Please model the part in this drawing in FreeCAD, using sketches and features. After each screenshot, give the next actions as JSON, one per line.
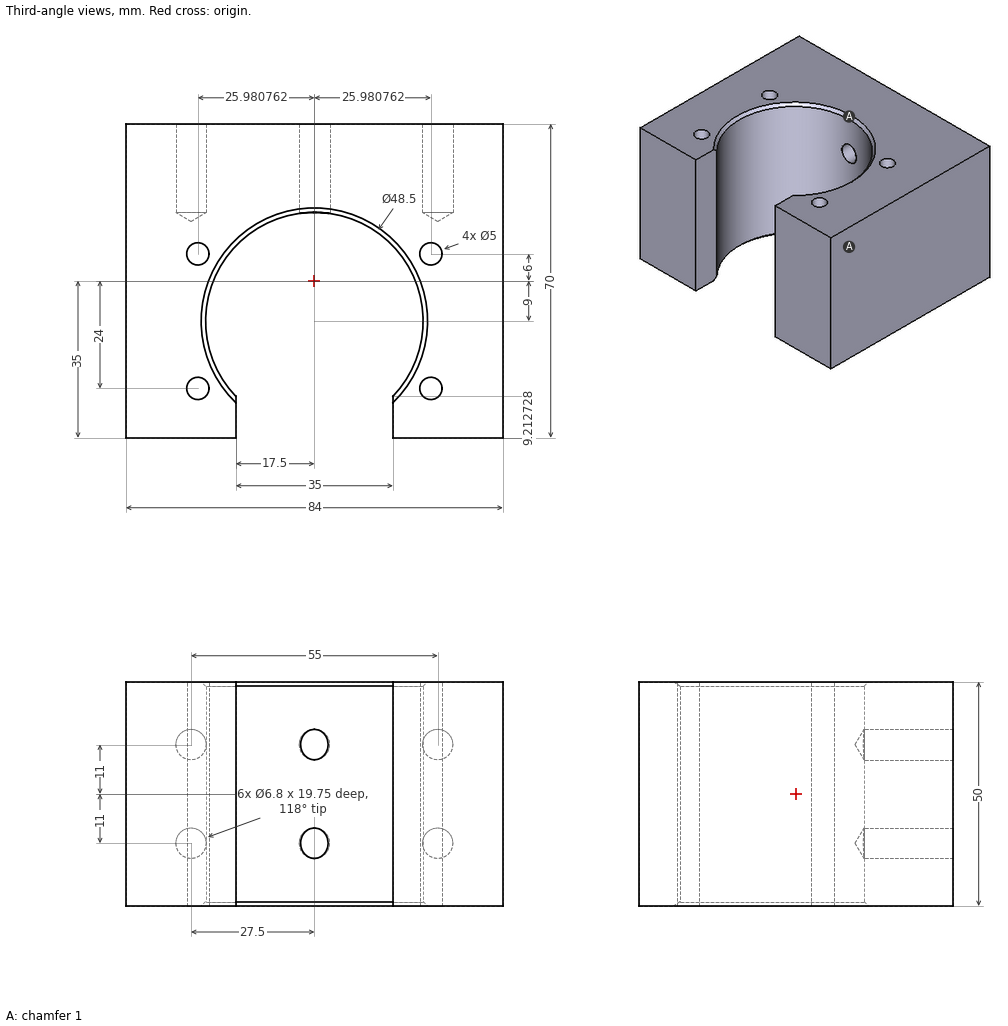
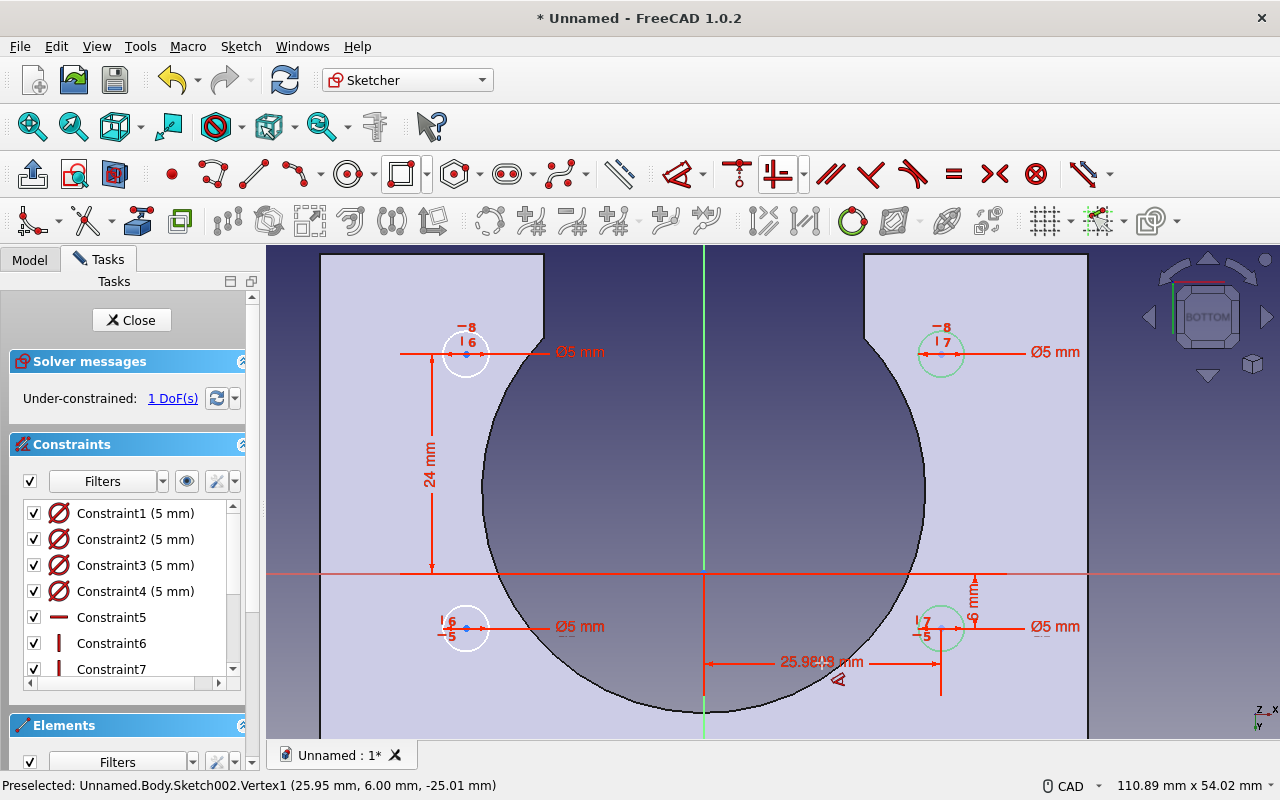
{"action": "left_click", "coordinate": [466, 629]}
{"action": "left_click", "coordinate": [585, 663]}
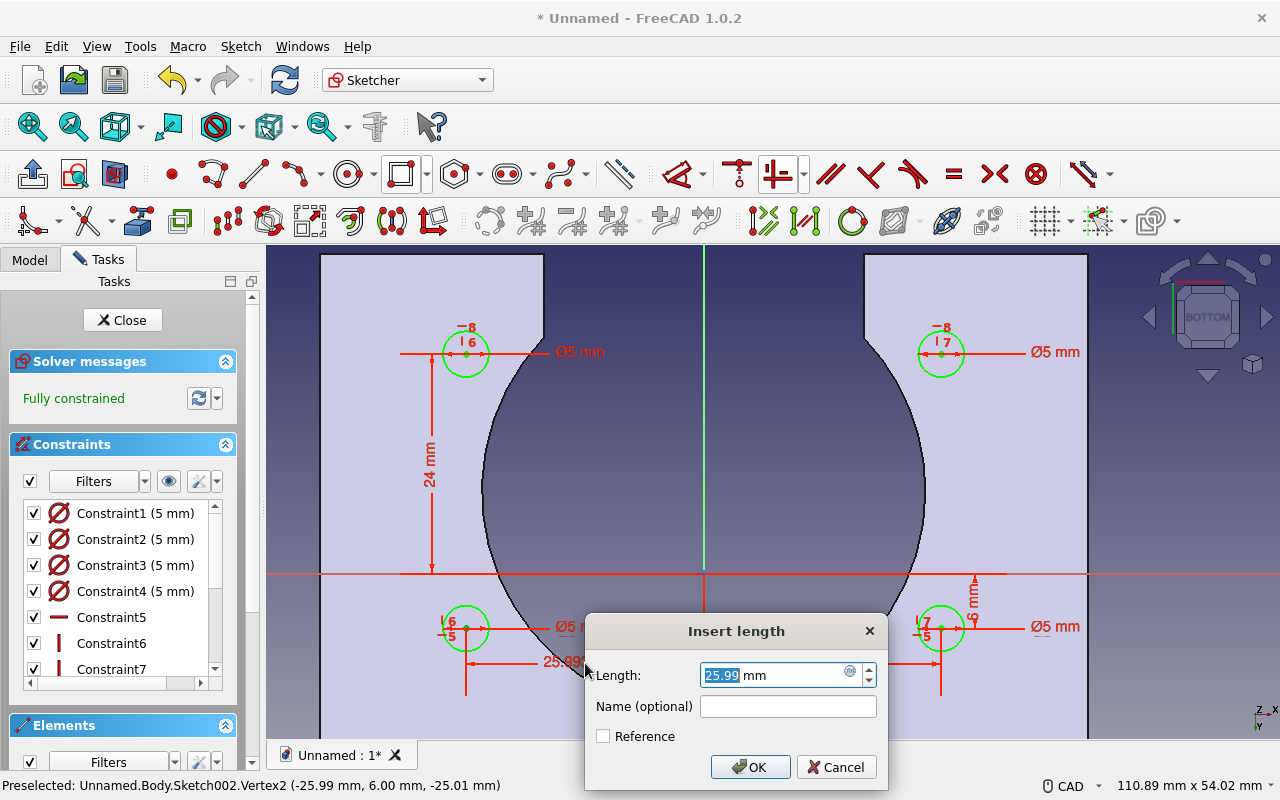
{"action": "type", "text": "25.980762"}
{"action": "key", "text": "Return"}
{"action": "key", "text": "Escape"}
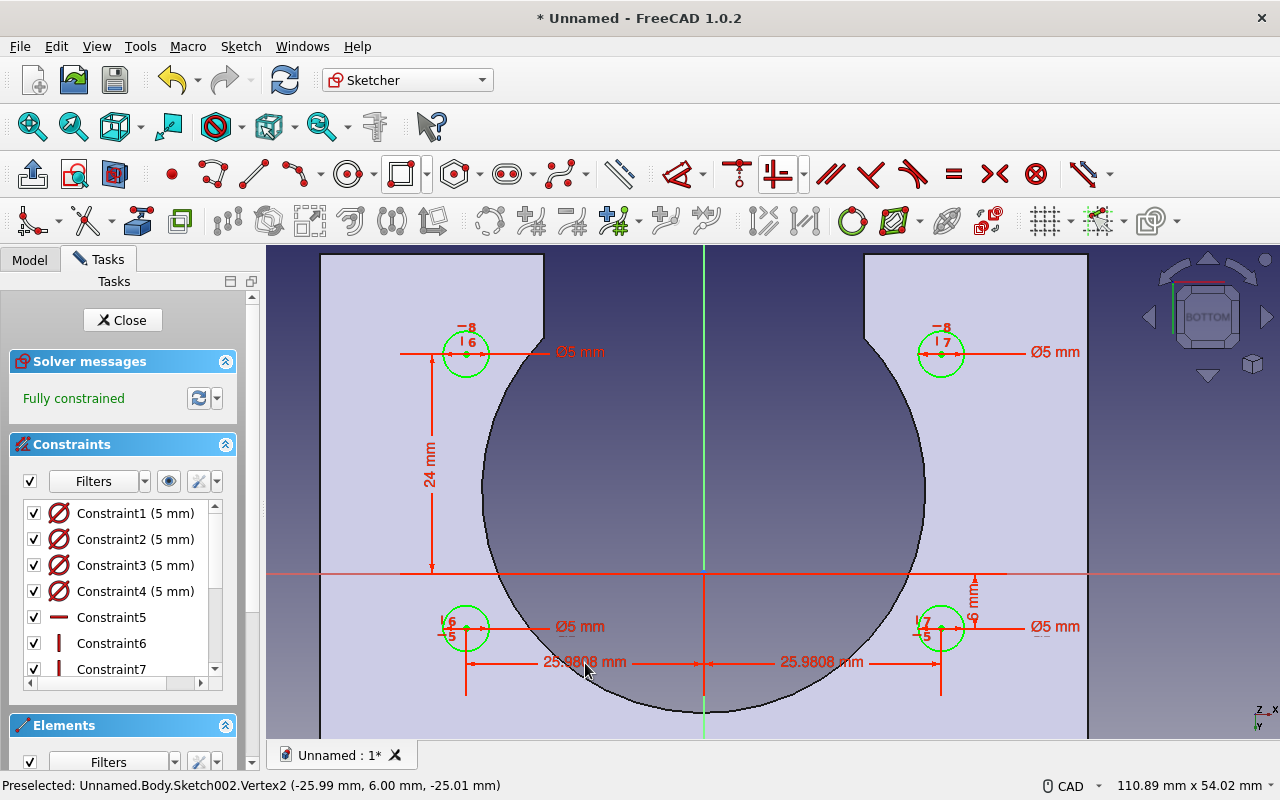
{"action": "left_click", "coordinate": [123, 320]}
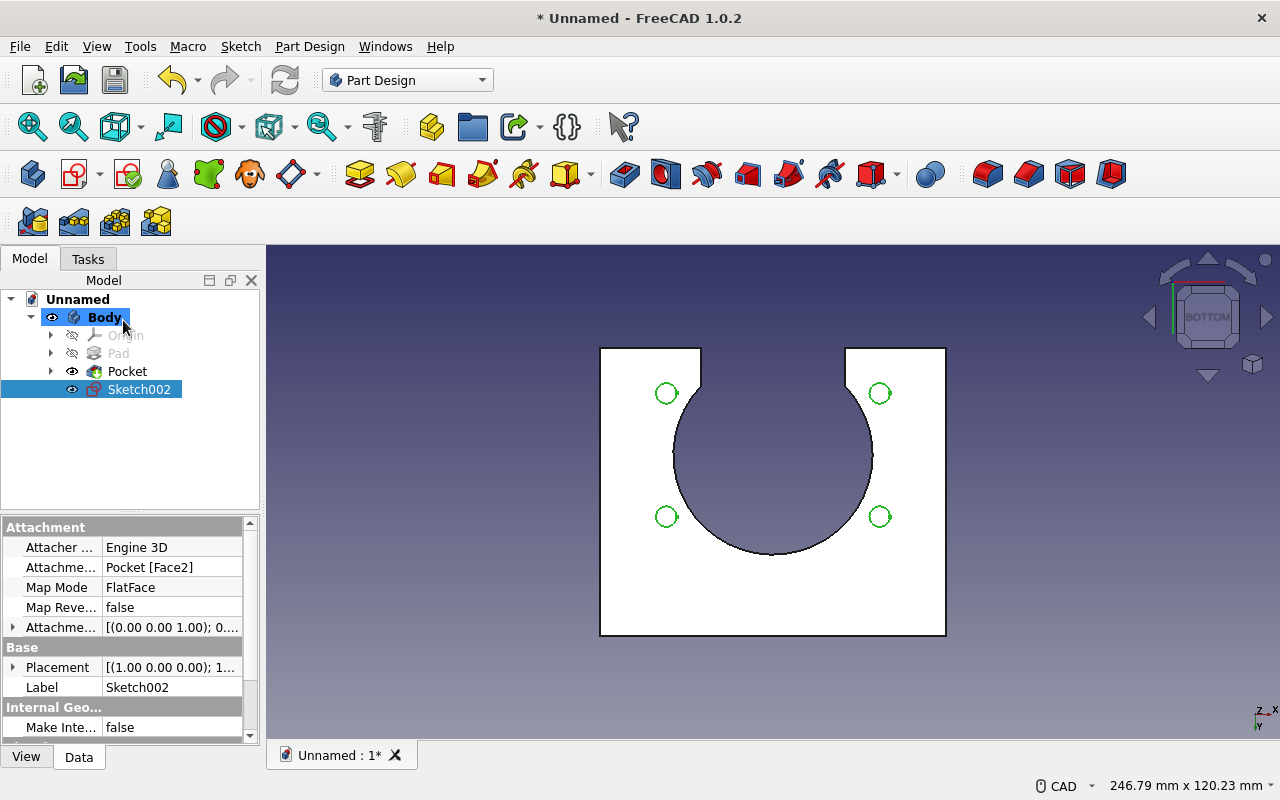
{"action": "left_click", "coordinate": [625, 174]}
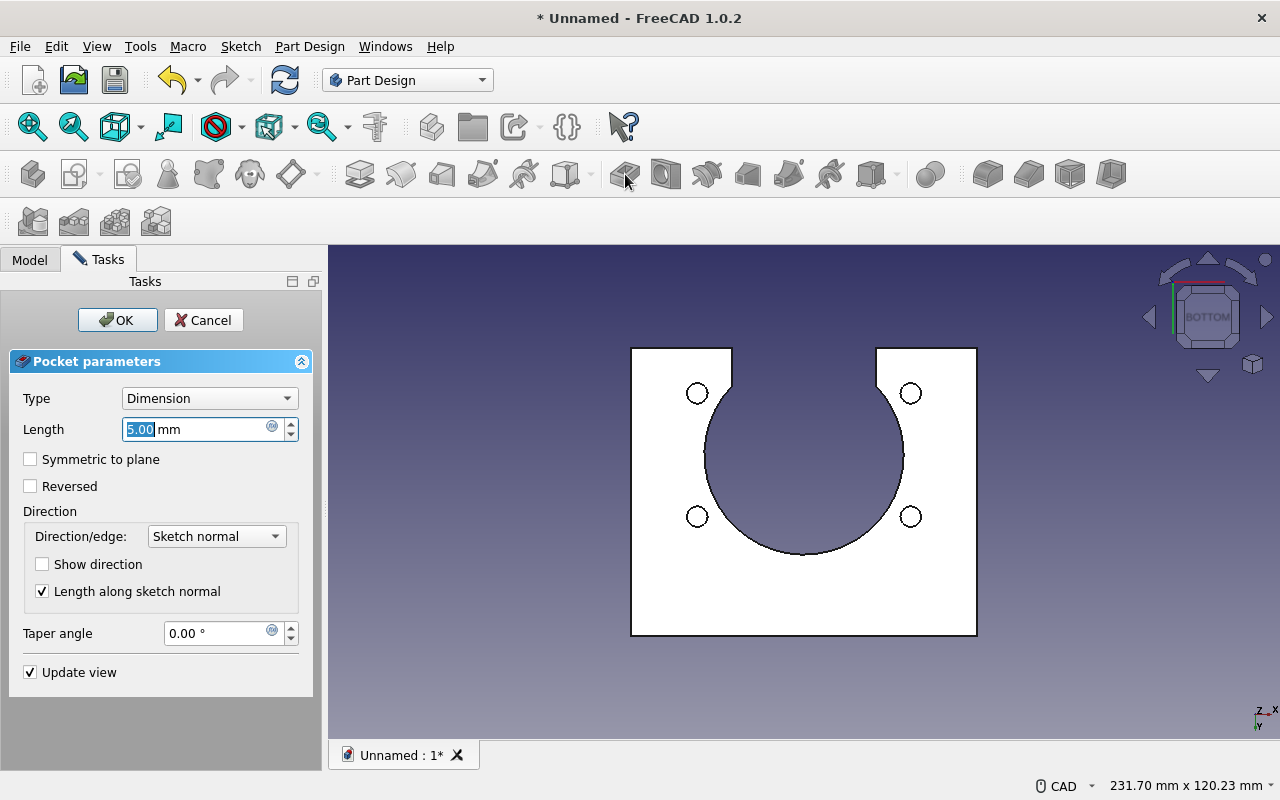
{"action": "left_click", "coordinate": [210, 398]}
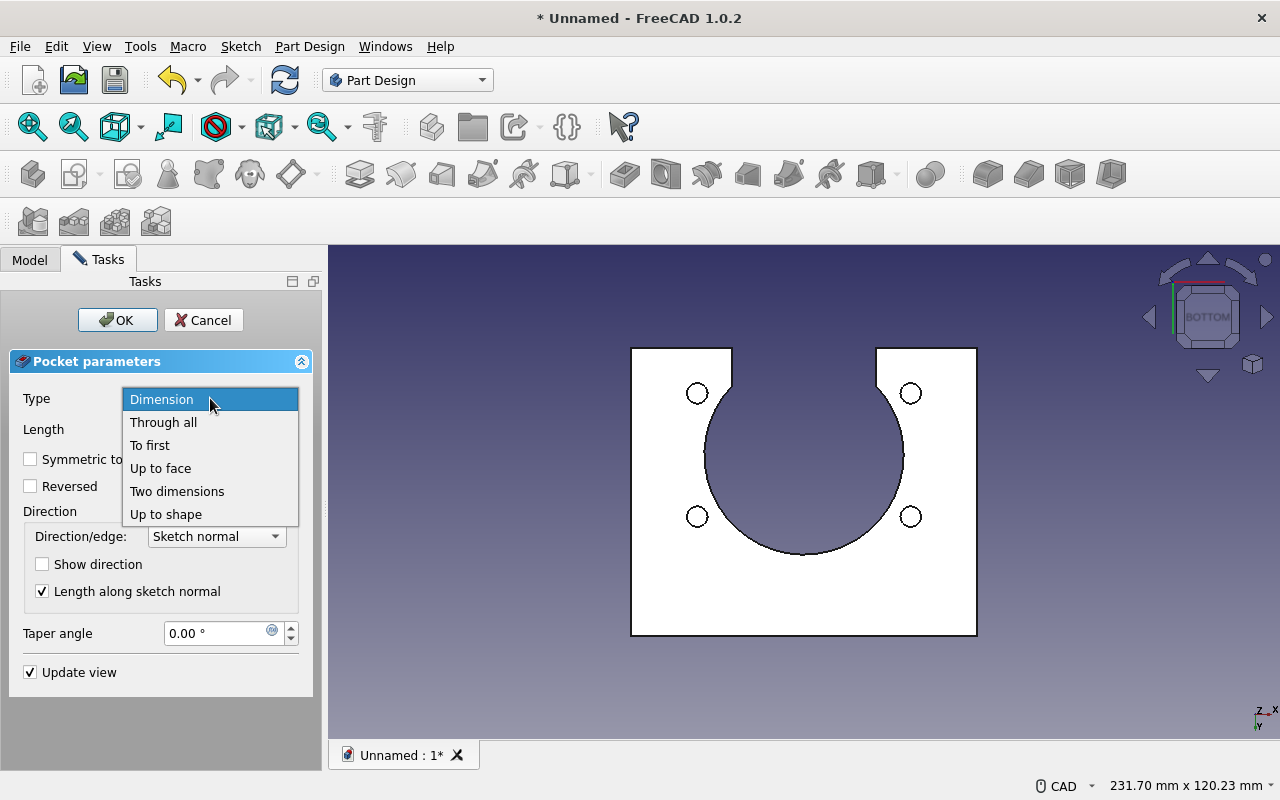
{"action": "left_click", "coordinate": [208, 422]}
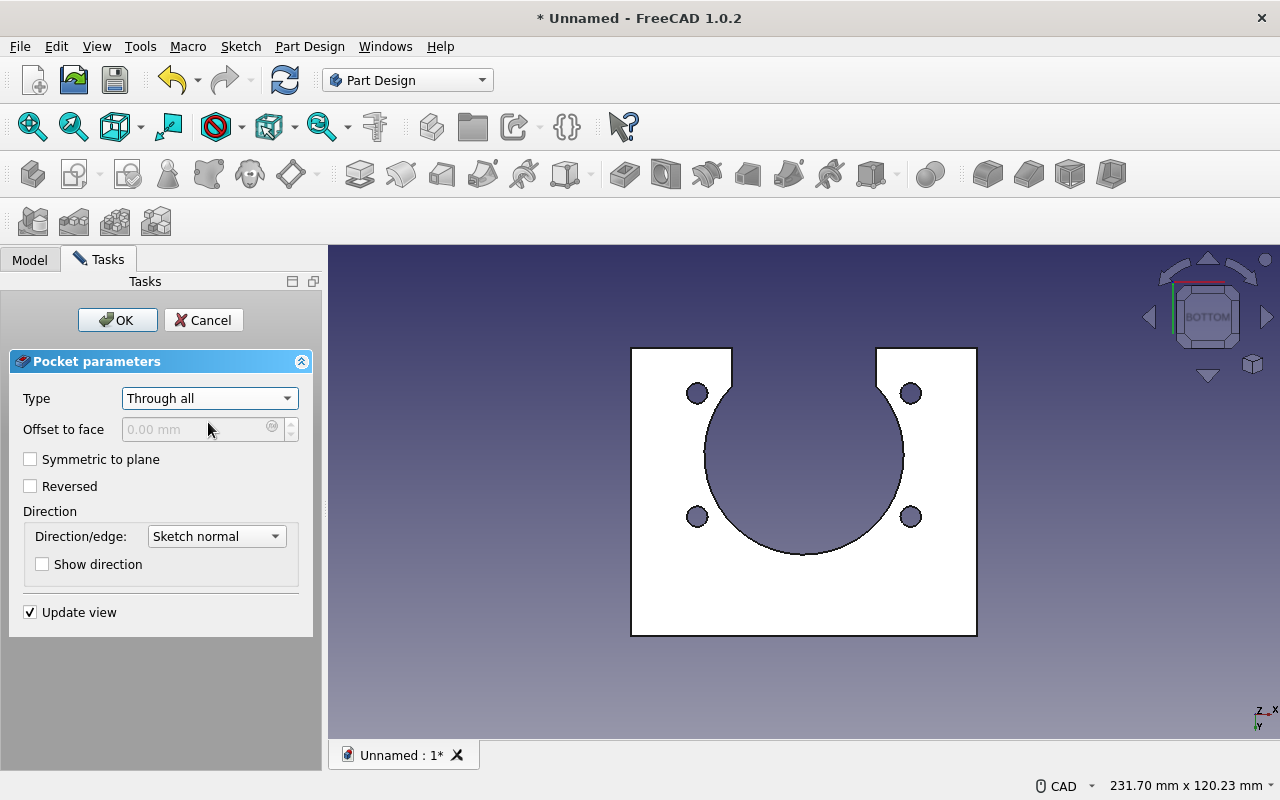
{"action": "left_click", "coordinate": [118, 320]}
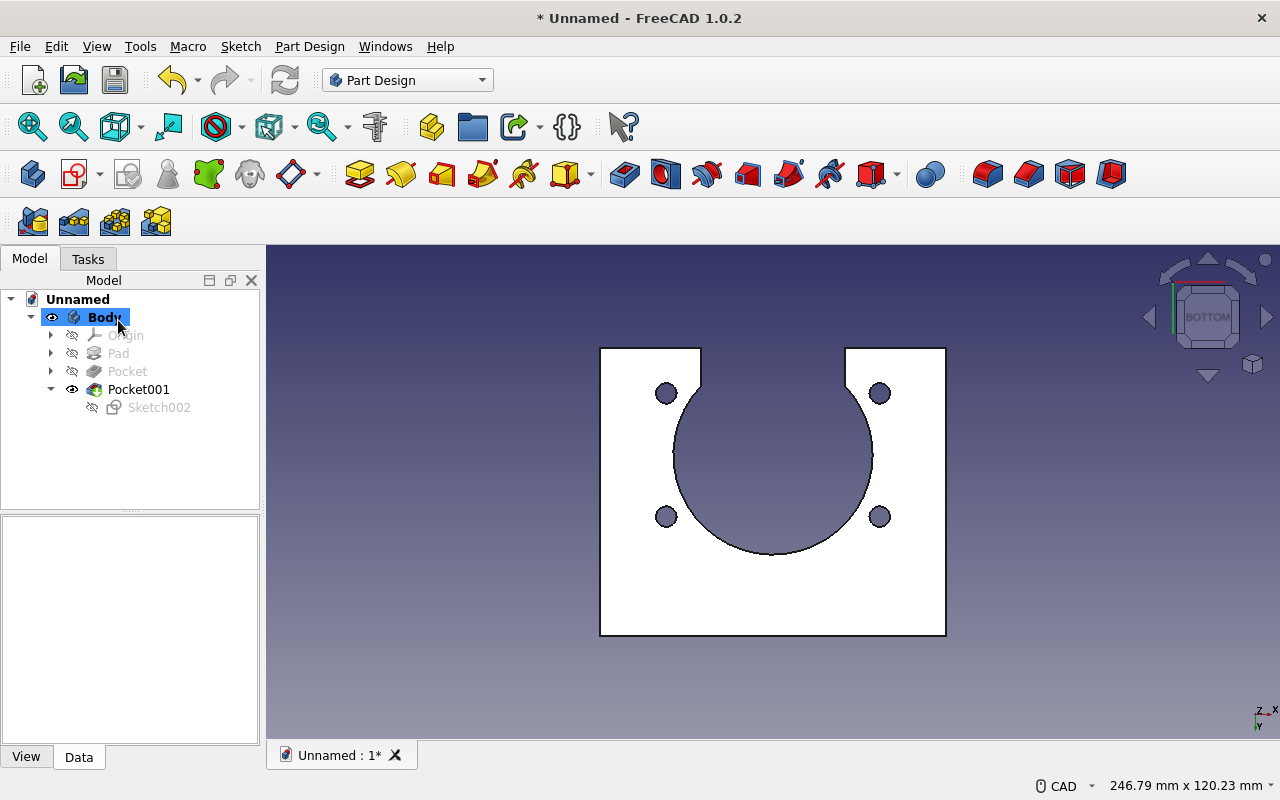
{"action": "key", "text": "4"}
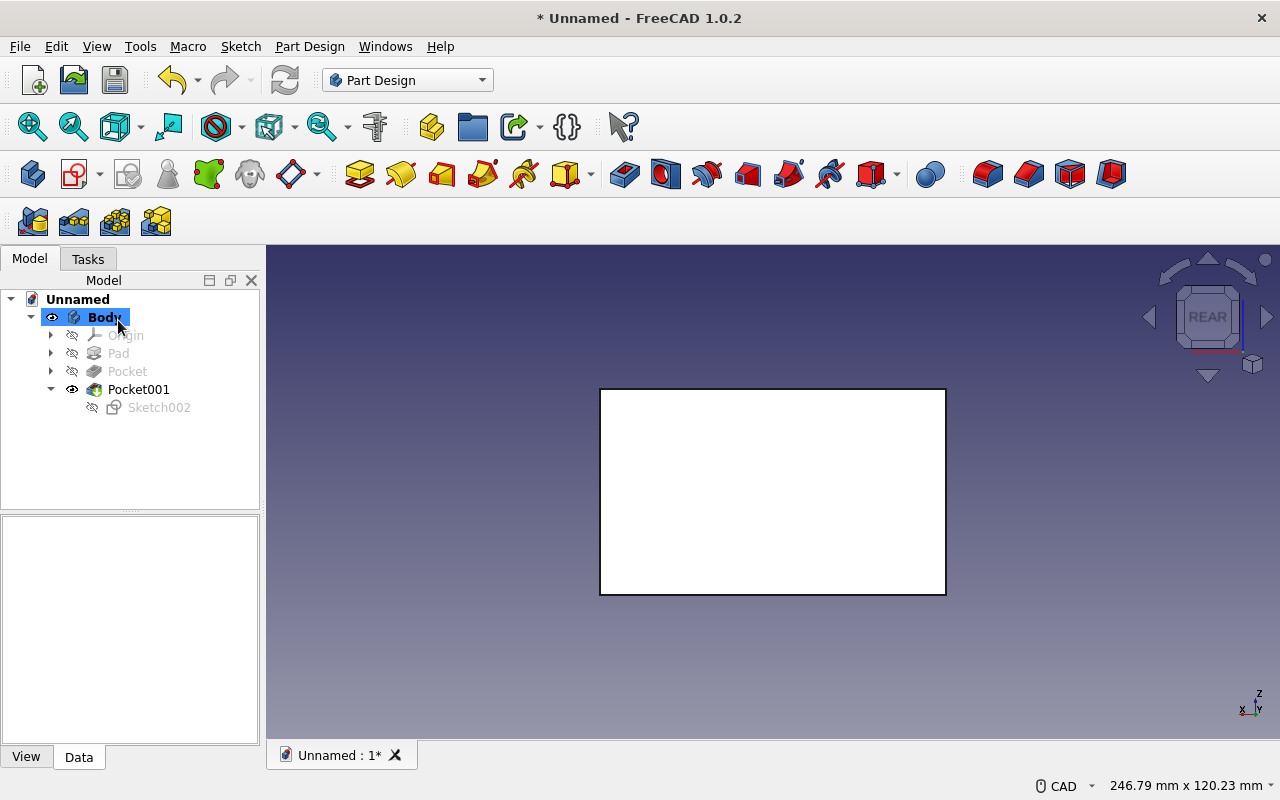
{"action": "left_click", "coordinate": [33, 128]}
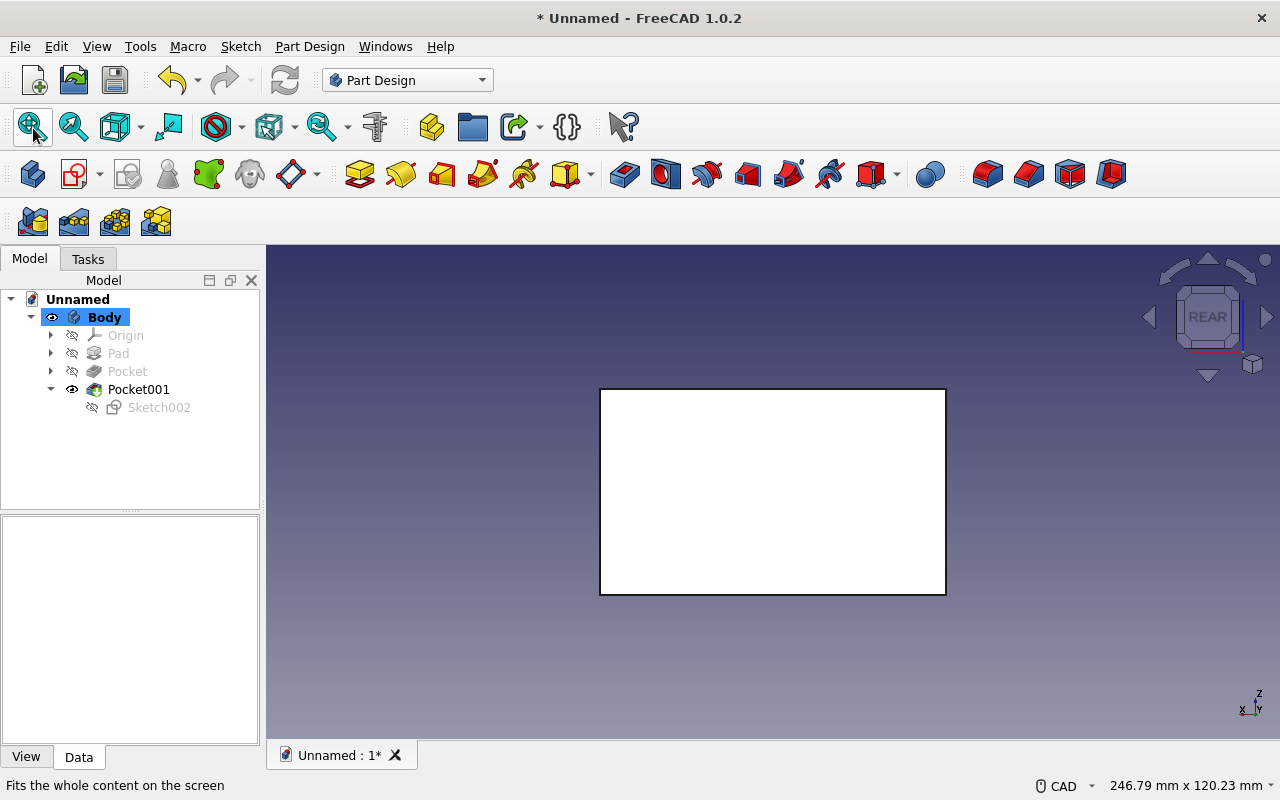
{"action": "left_click", "coordinate": [724, 491]}